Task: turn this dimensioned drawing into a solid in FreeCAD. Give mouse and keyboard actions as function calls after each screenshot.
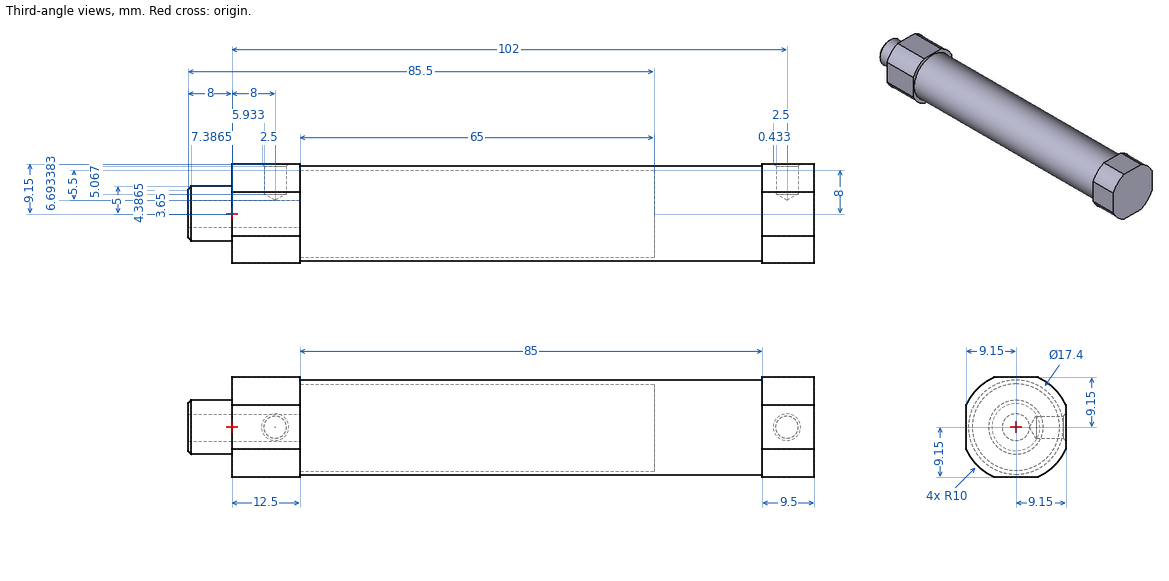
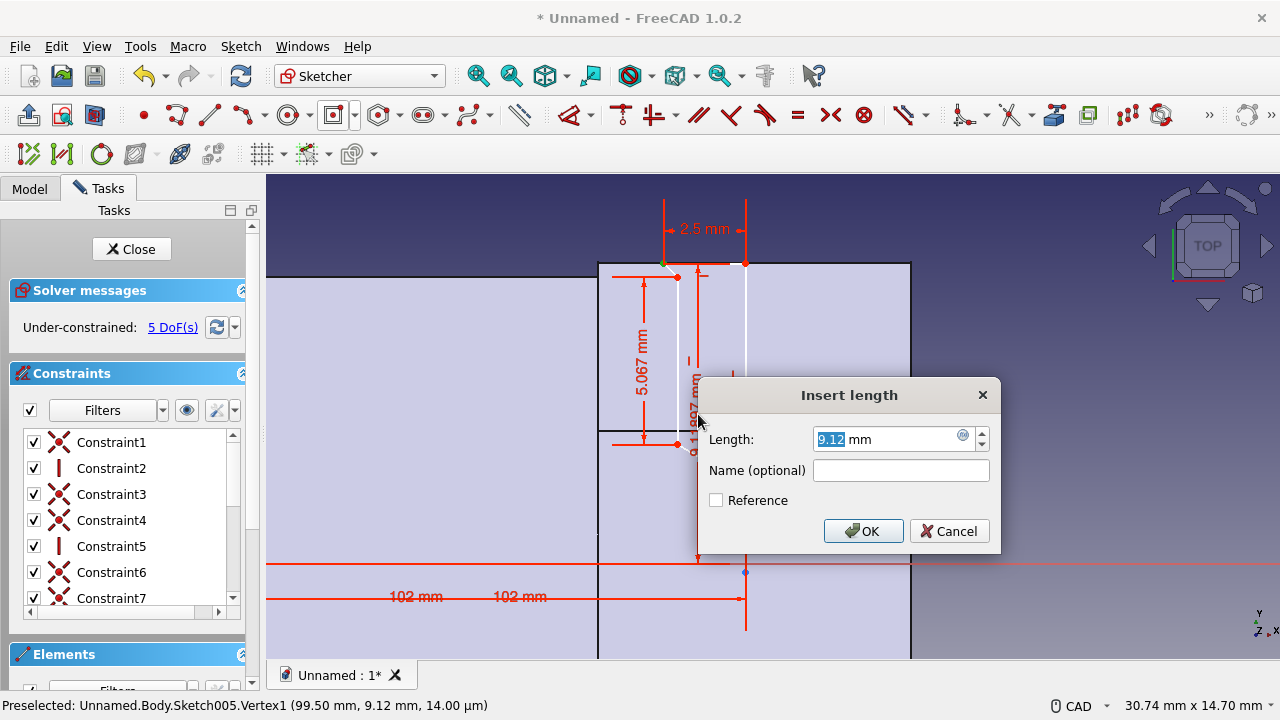
text(9.15)
key(Return)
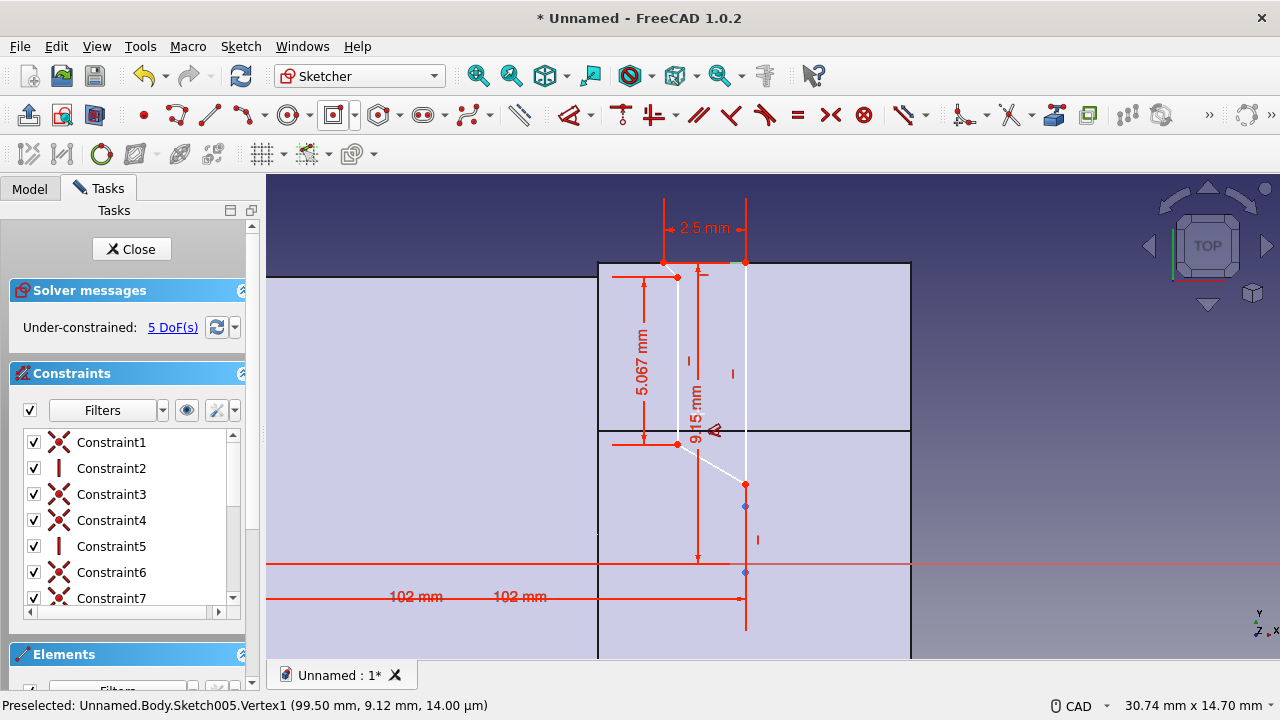
click(678, 445)
click(712, 504)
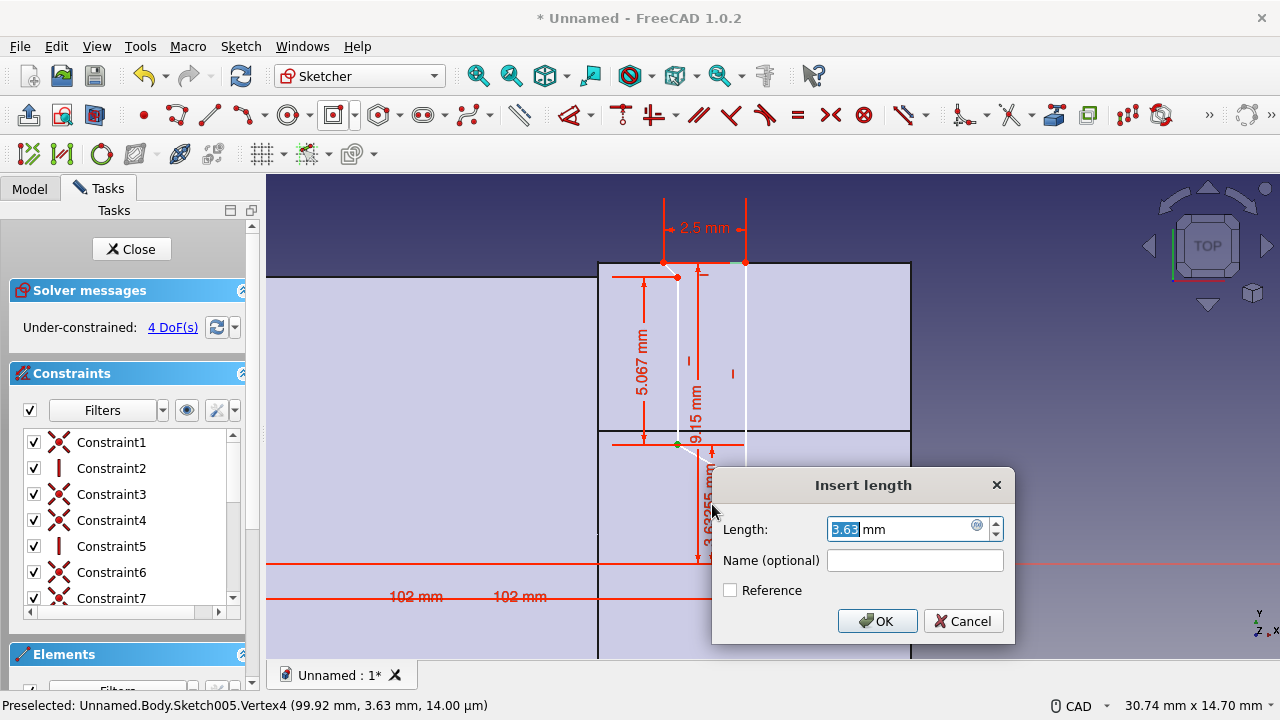
text(3.65)
key(Return)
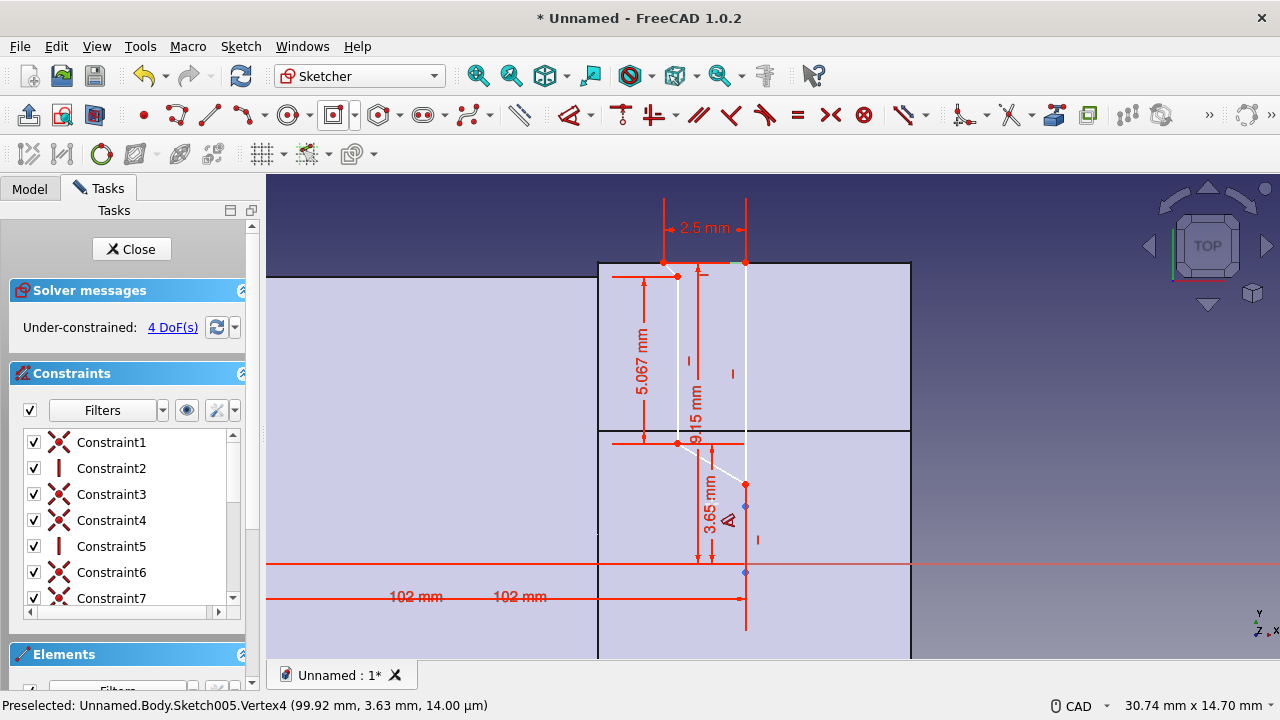
scroll(672, 271, up, 6)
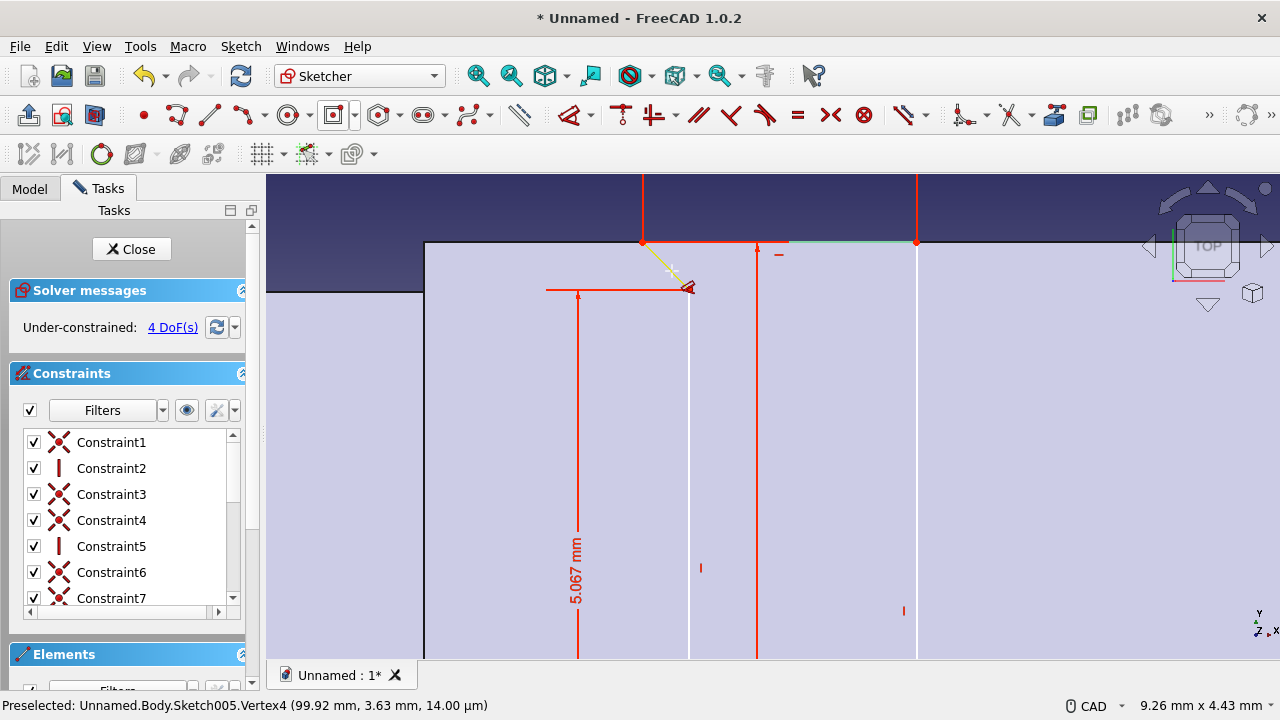
click(671, 271)
click(666, 208)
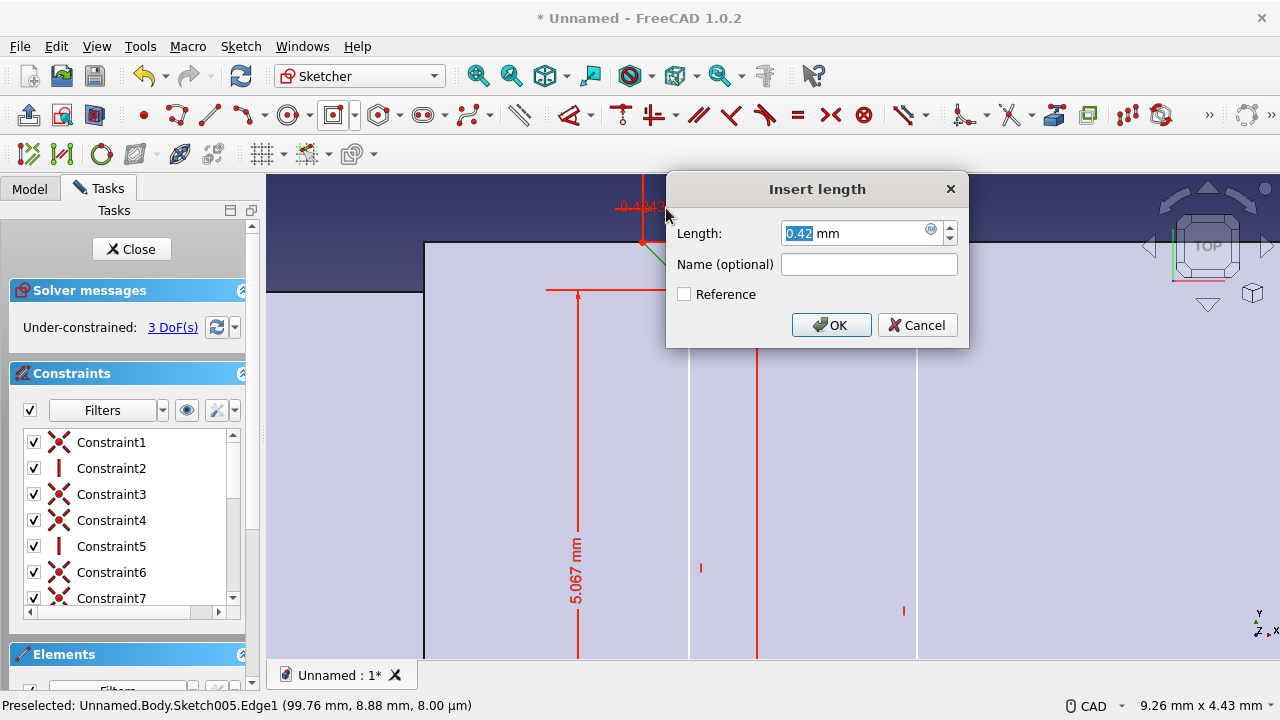
text(0.433)
key(Return)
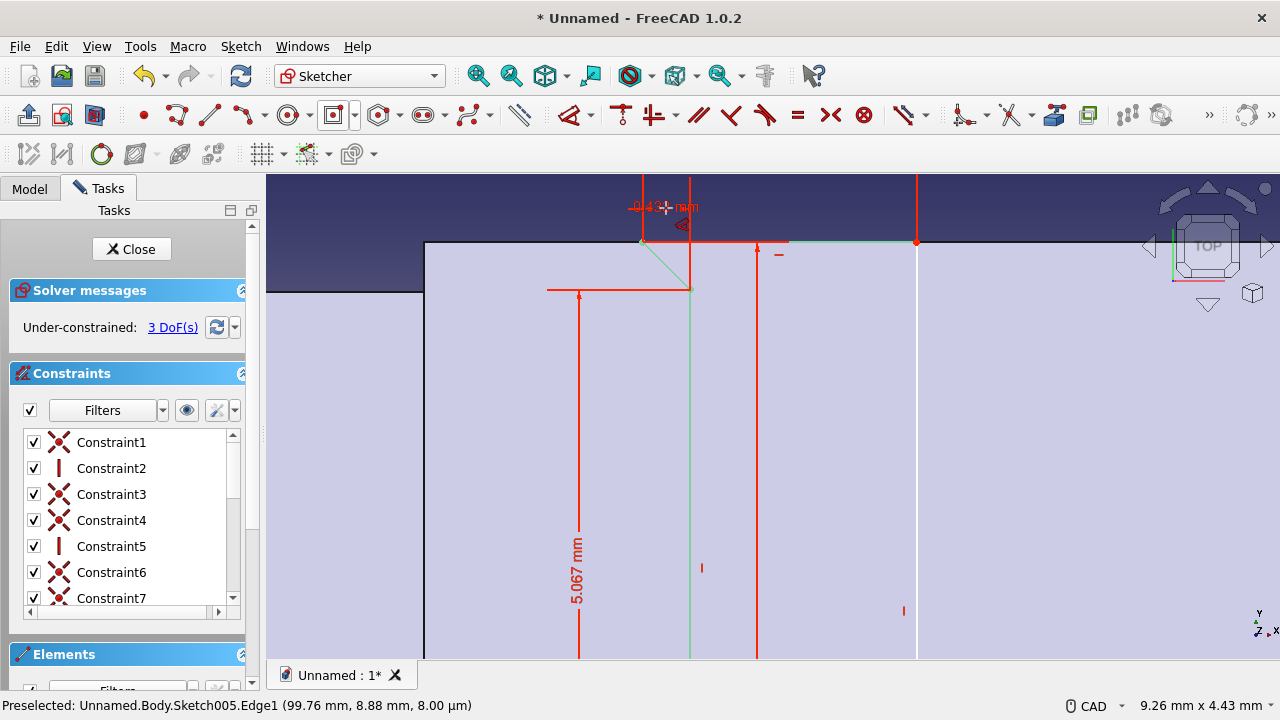
click(917, 463)
click(951, 437)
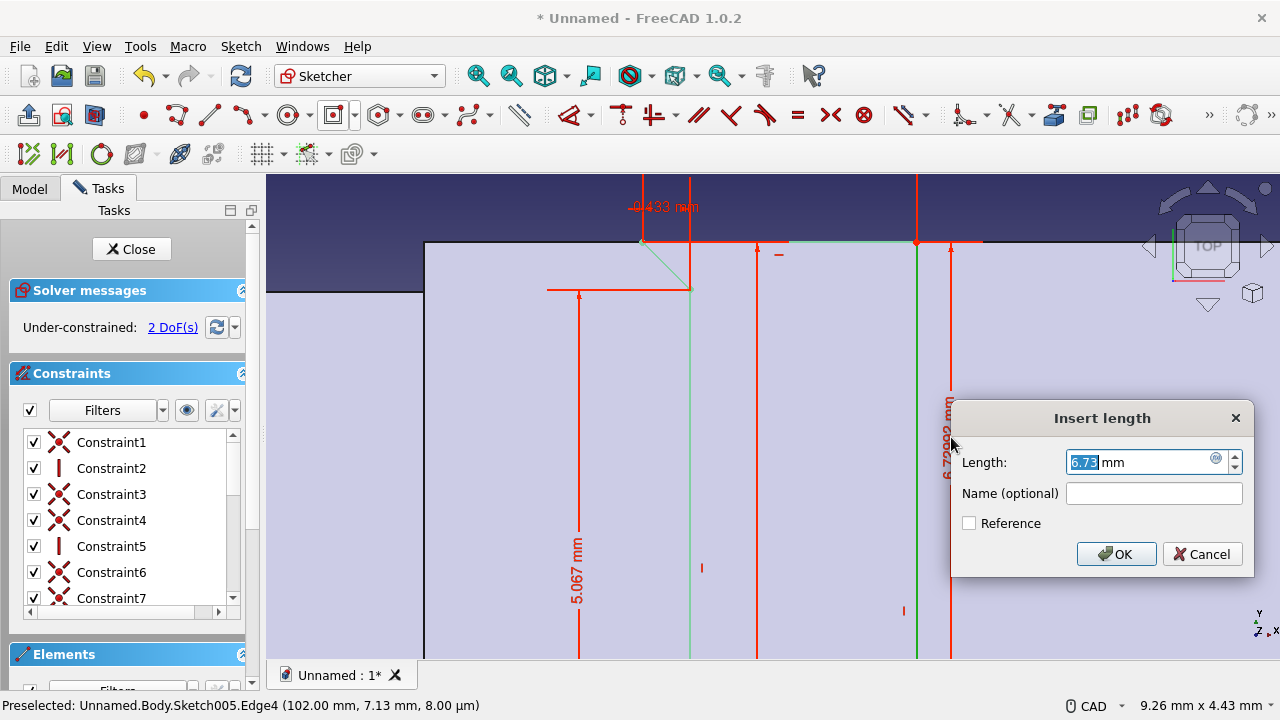
text(6.693383)
key(Return)
key(Escape)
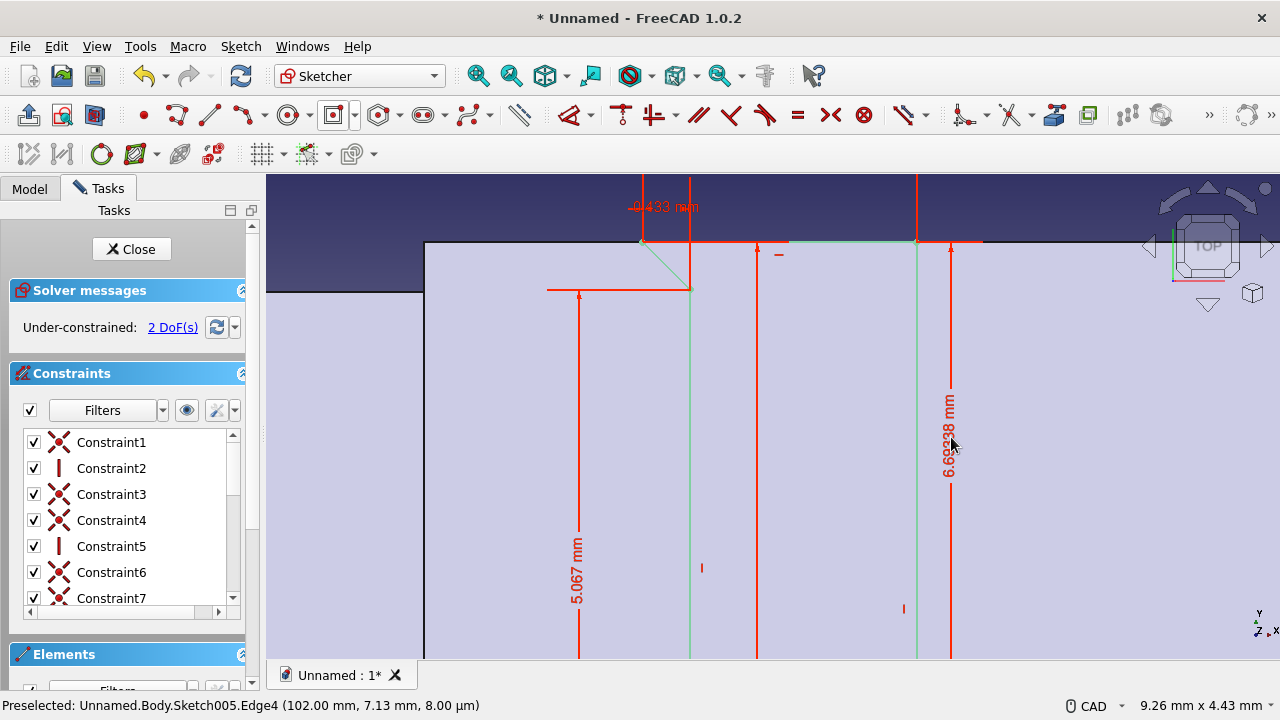
click(132, 249)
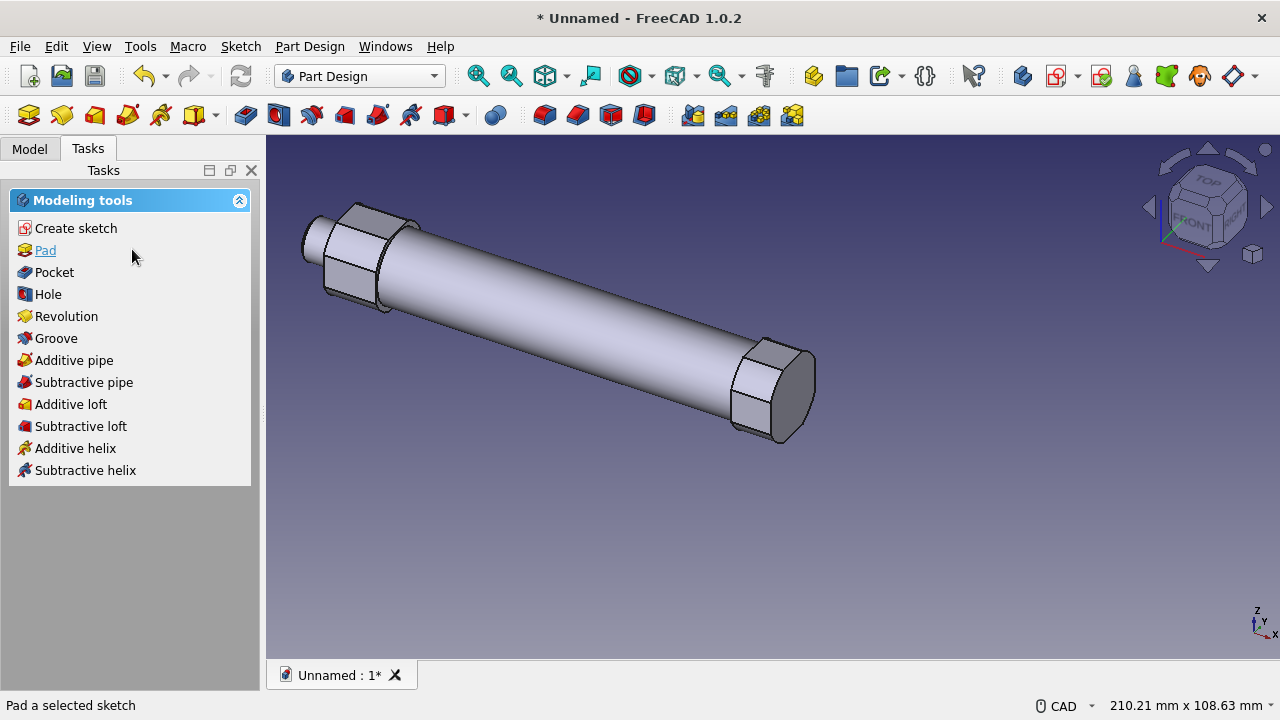
click(312, 116)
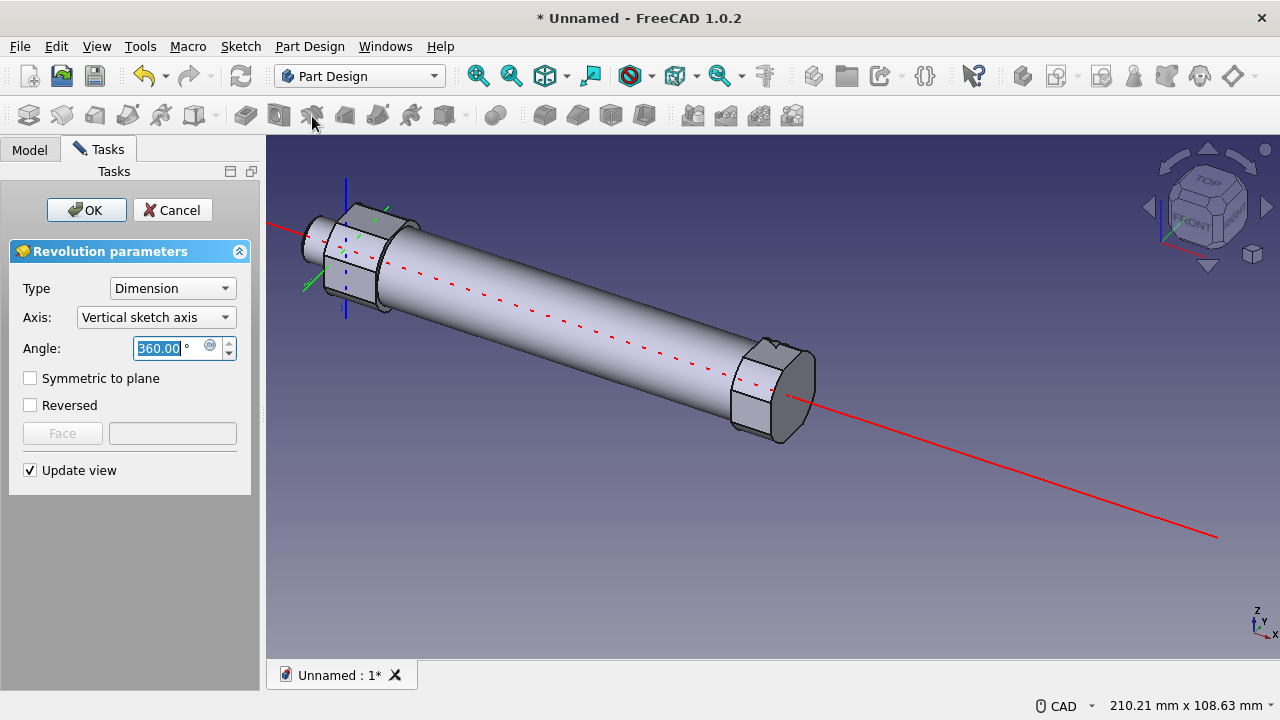
click(157, 318)